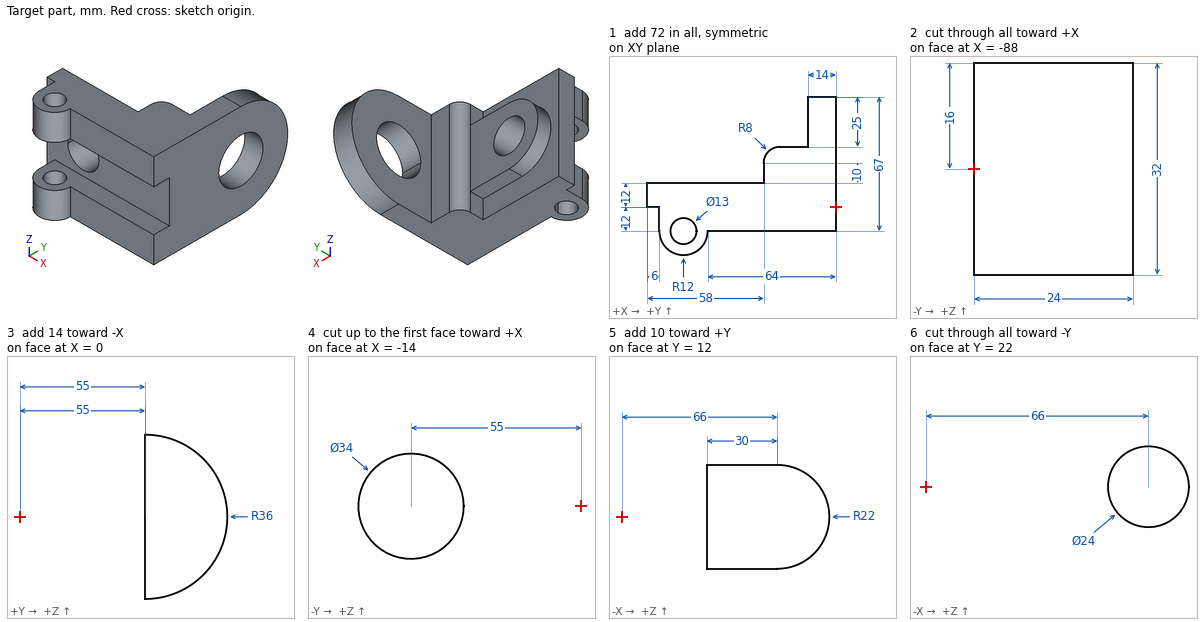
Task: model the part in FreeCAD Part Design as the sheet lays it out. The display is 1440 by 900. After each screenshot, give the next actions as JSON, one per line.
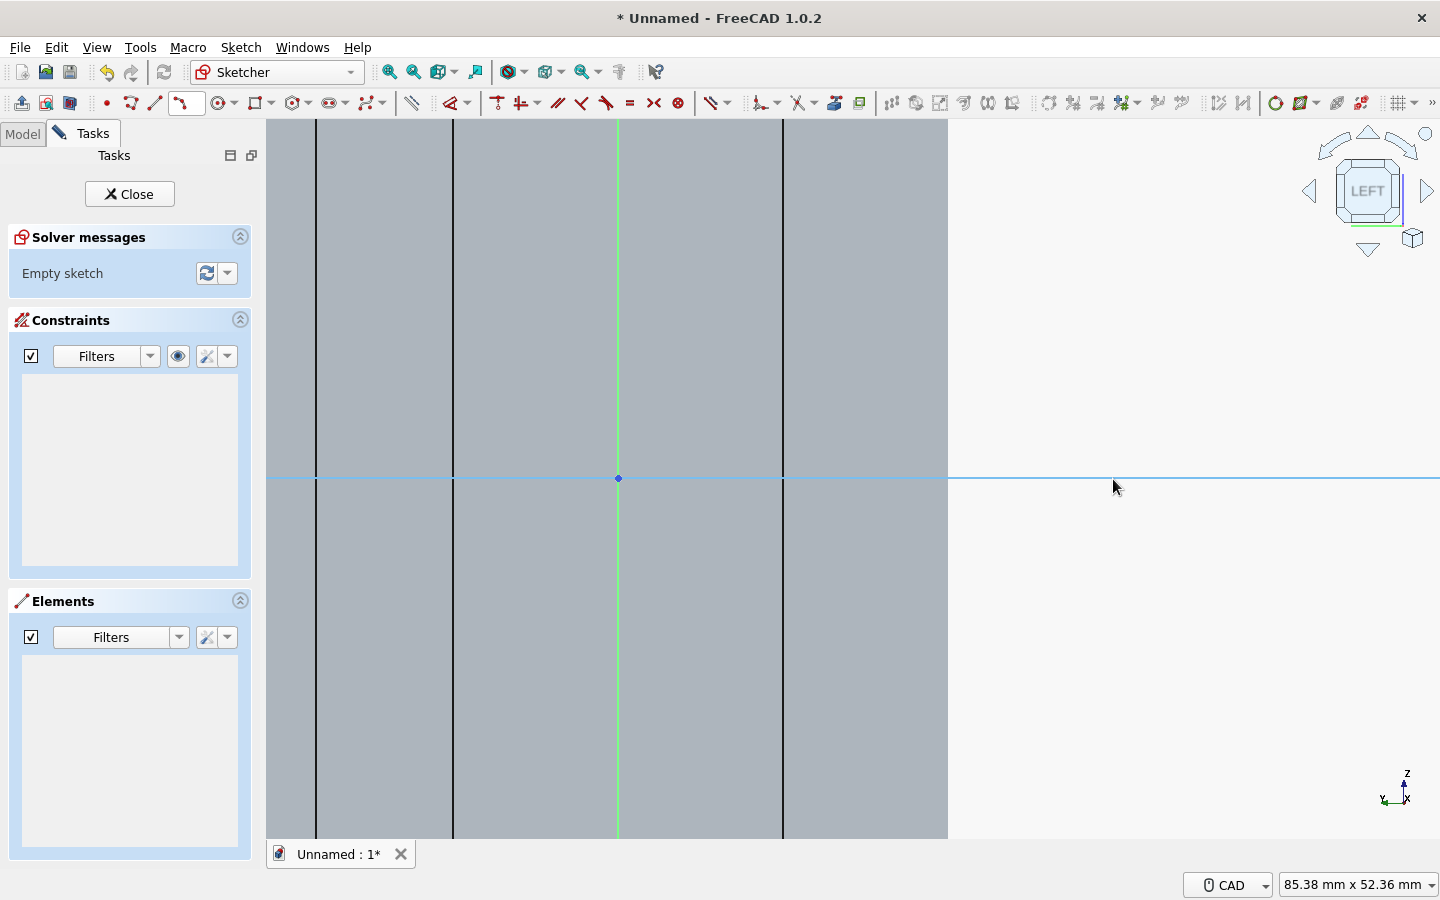
{"action": "left_click", "coordinate": [256, 104]}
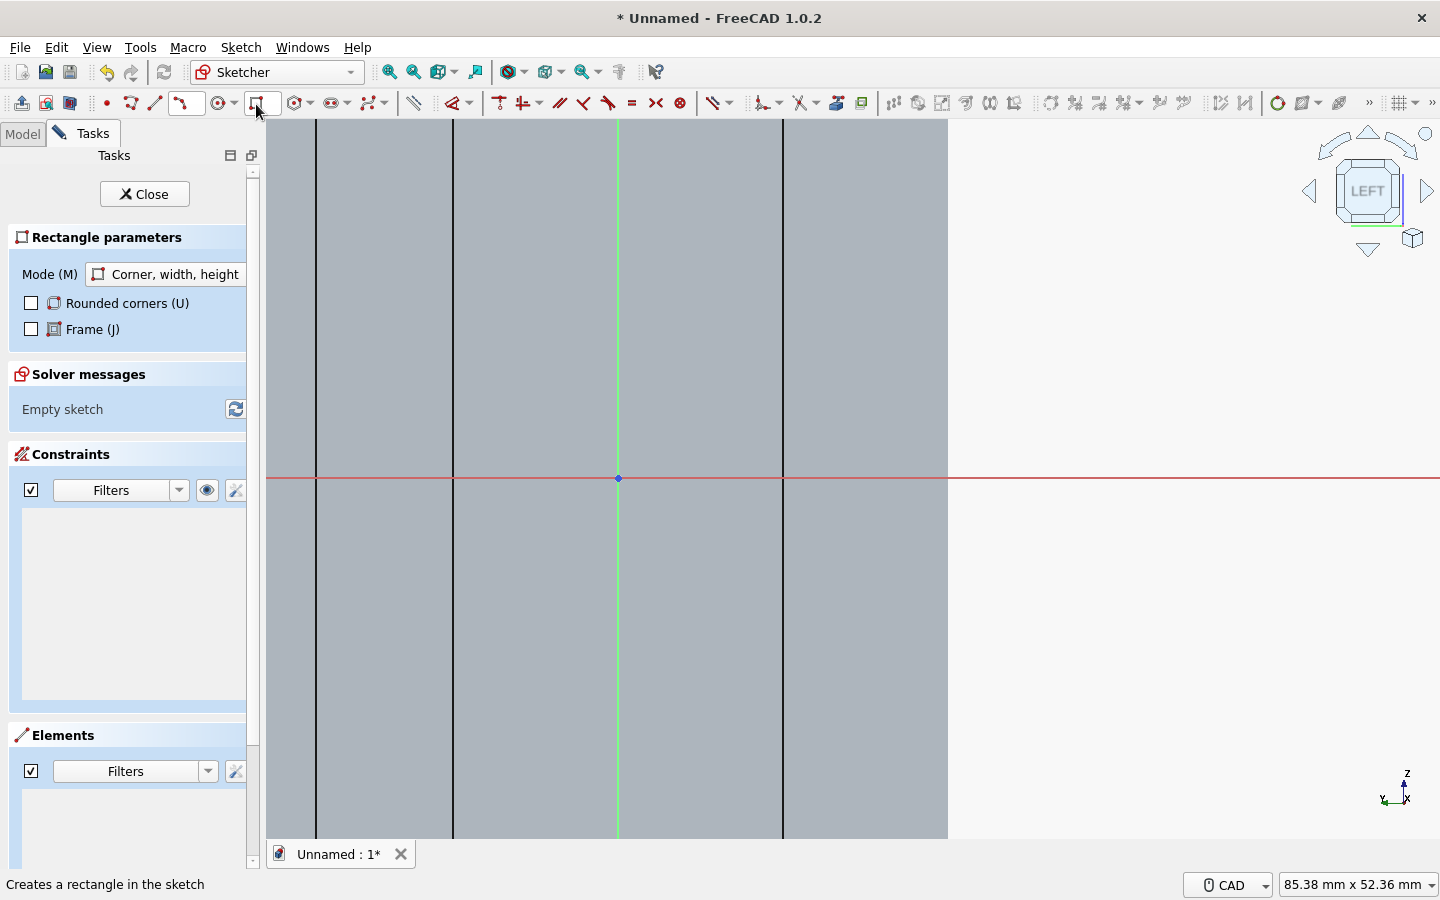
{"action": "left_click", "coordinate": [618, 258]}
{"action": "mouse_move", "coordinate": [948, 698]}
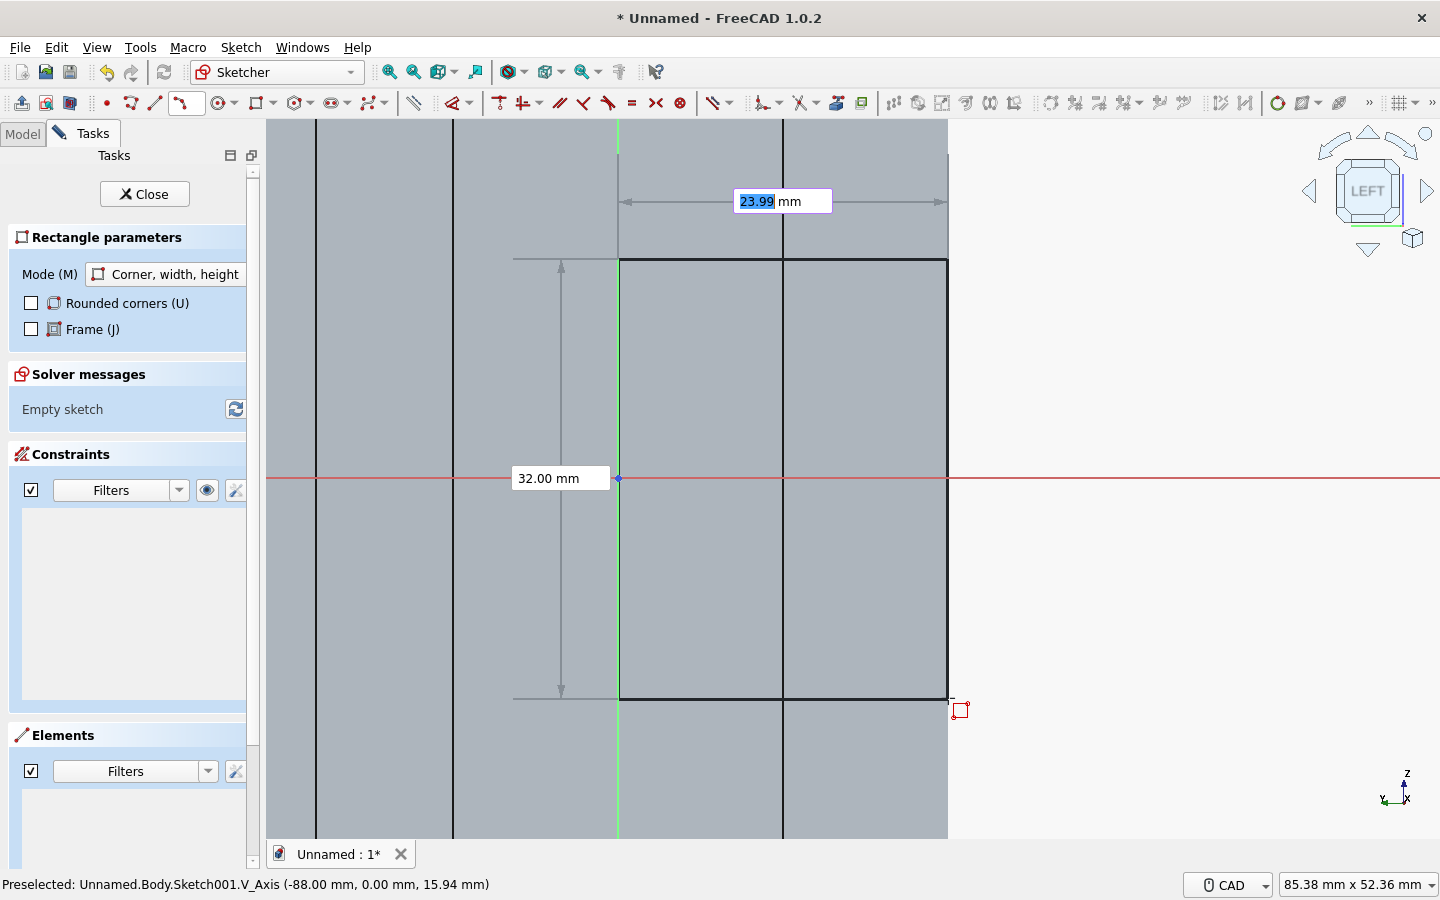
{"action": "type", "text": "24"}
{"action": "key", "text": "Tab"}
{"action": "type", "text": "32"}
{"action": "key", "text": "Return"}
{"action": "key", "text": "Escape"}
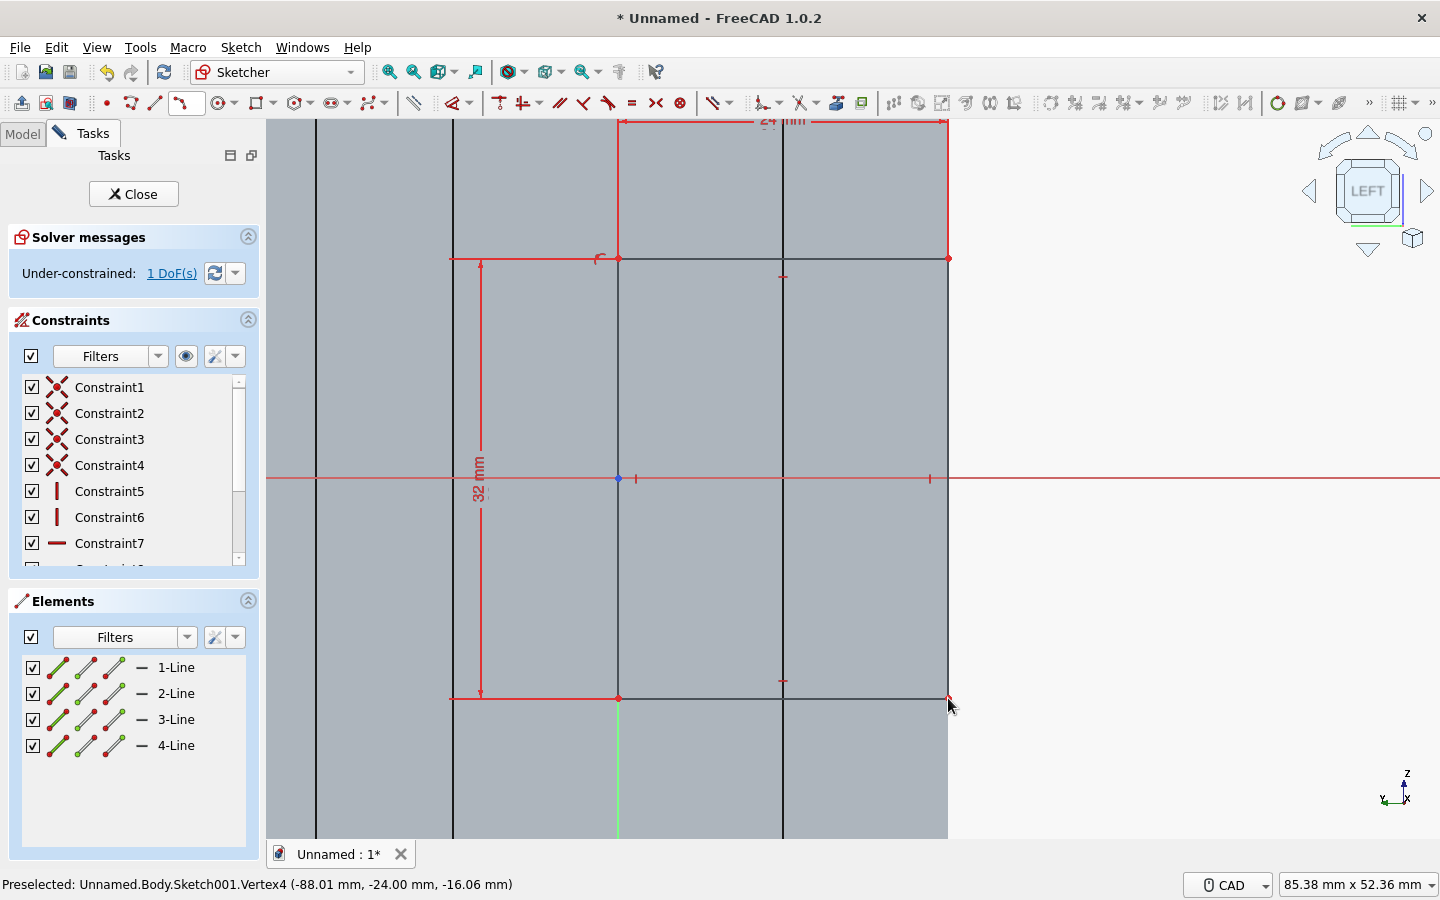
{"action": "left_click", "coordinate": [452, 104]}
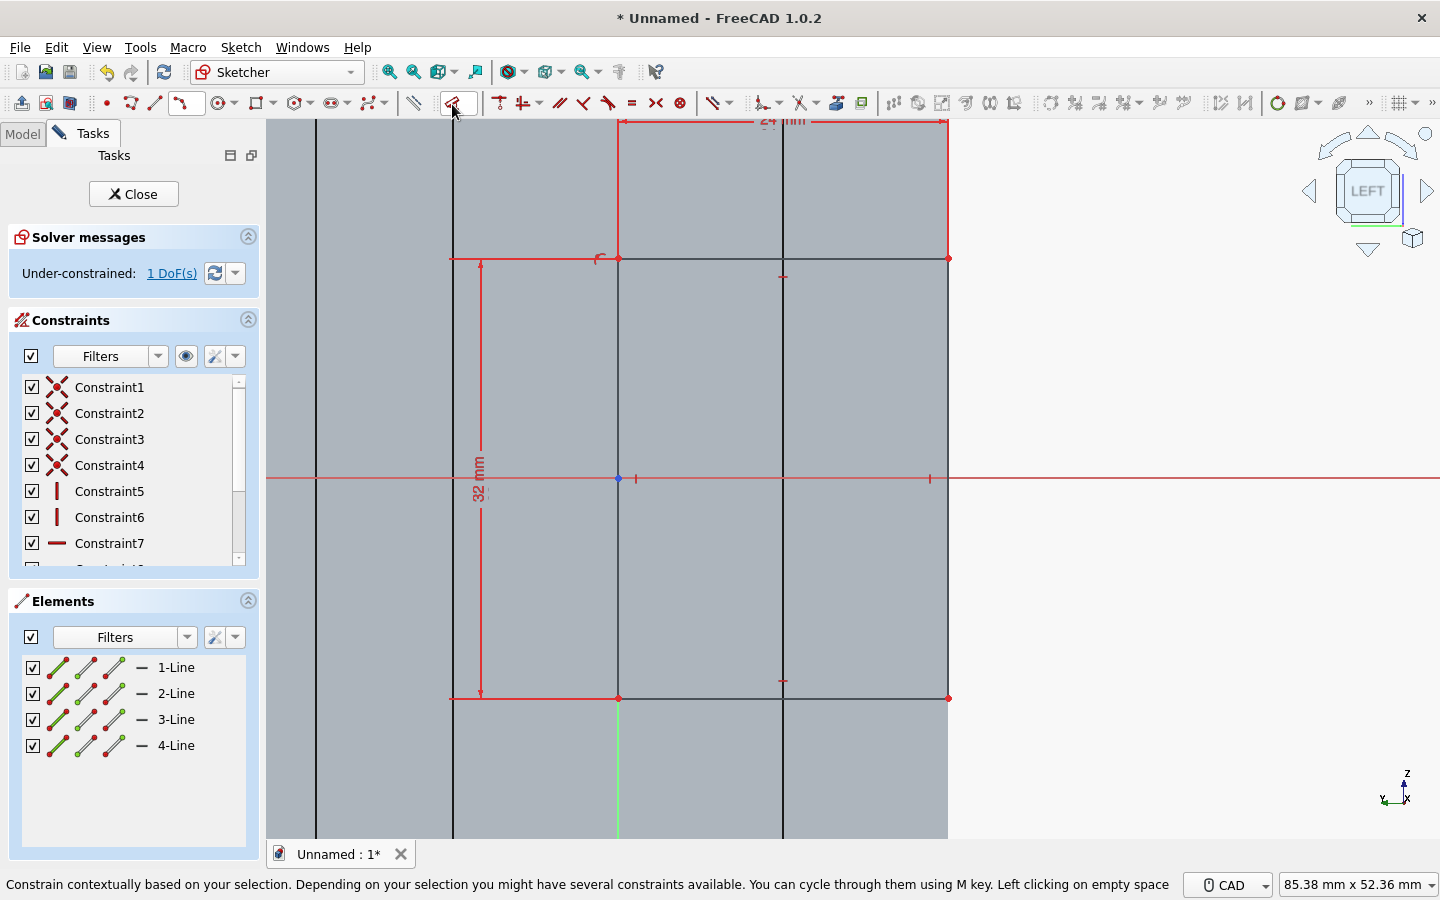
{"action": "left_click", "coordinate": [618, 259]}
{"action": "left_click", "coordinate": [584, 369]}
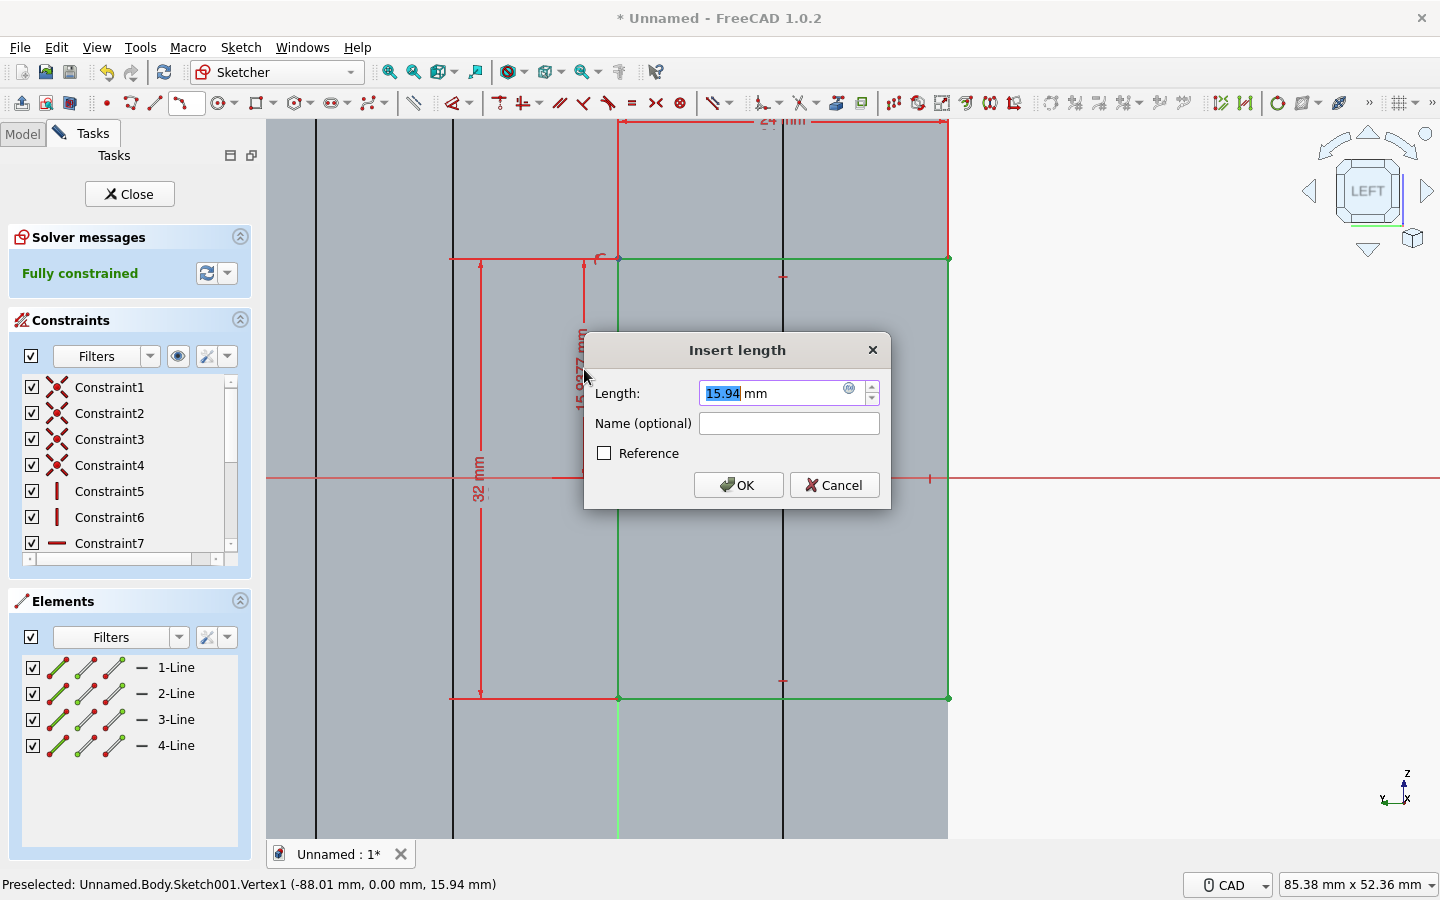
{"action": "type", "text": "16"}
{"action": "key", "text": "Return"}
{"action": "key", "text": "Escape"}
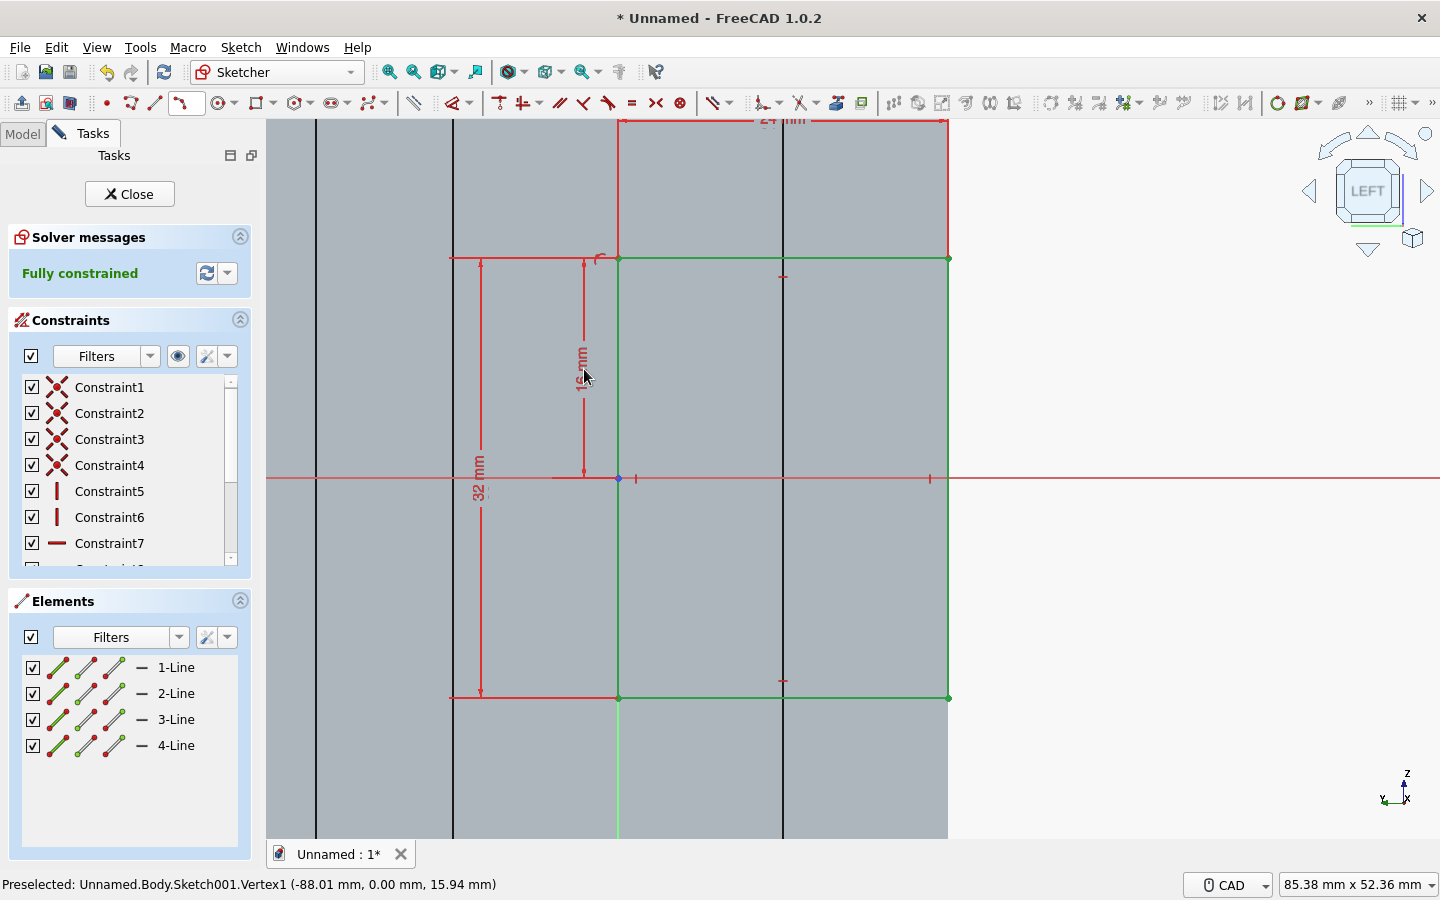
{"action": "left_click", "coordinate": [130, 194]}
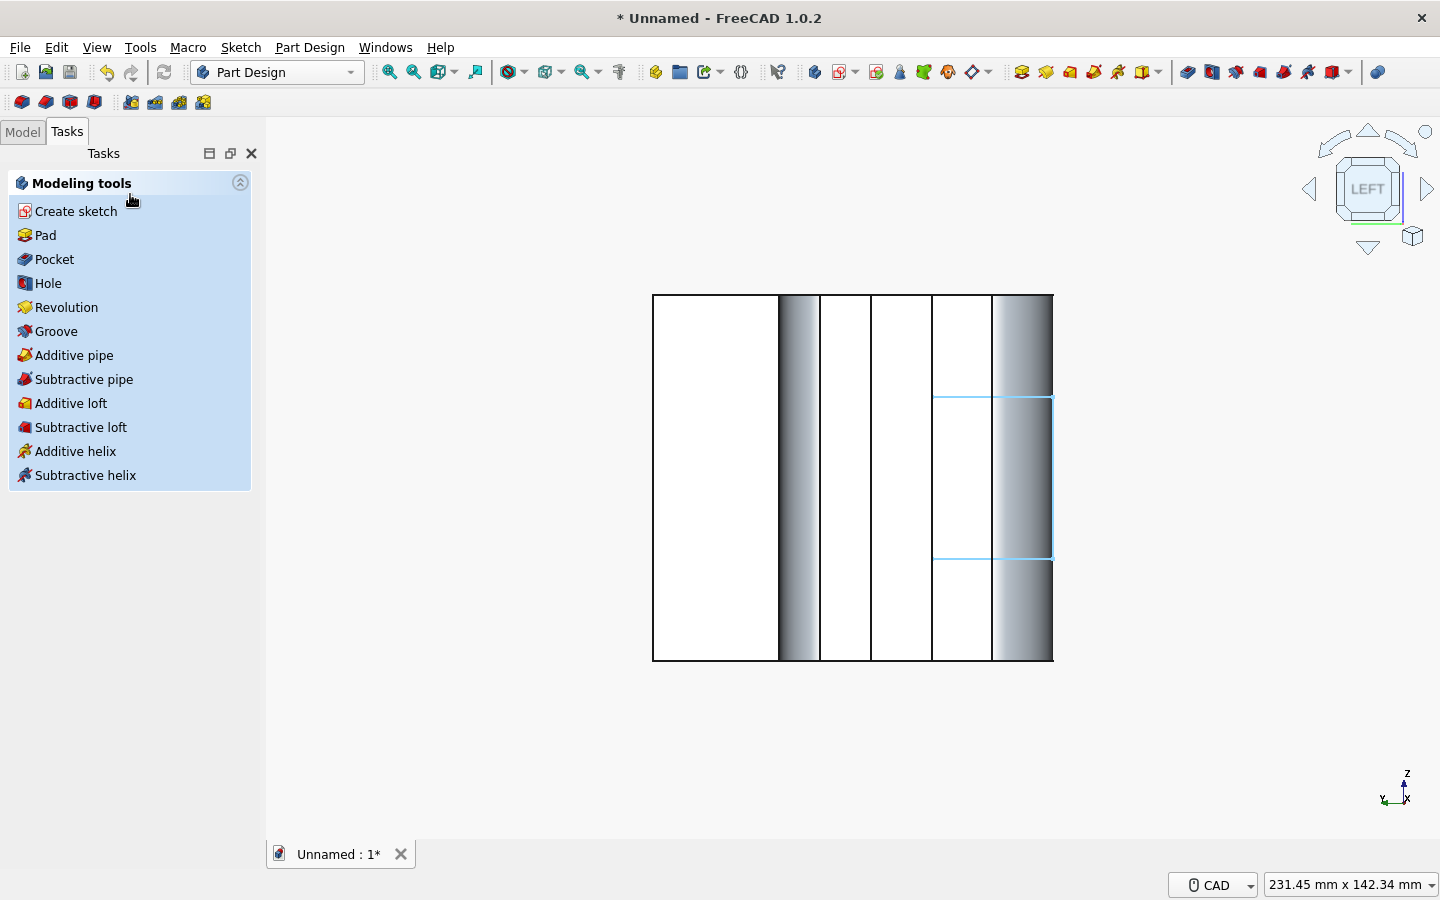
{"action": "left_click", "coordinate": [1188, 72]}